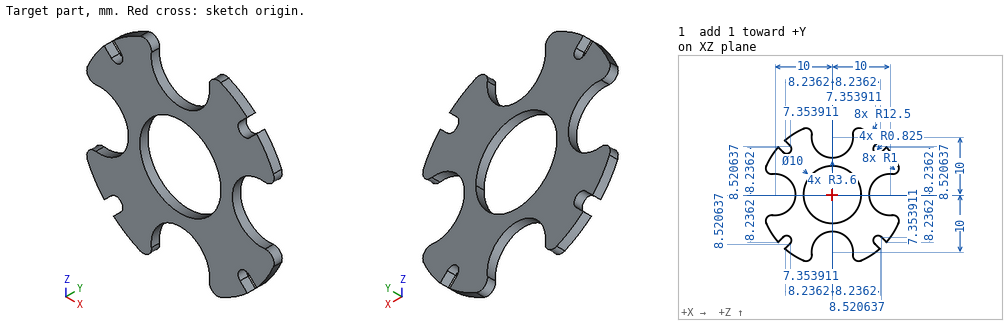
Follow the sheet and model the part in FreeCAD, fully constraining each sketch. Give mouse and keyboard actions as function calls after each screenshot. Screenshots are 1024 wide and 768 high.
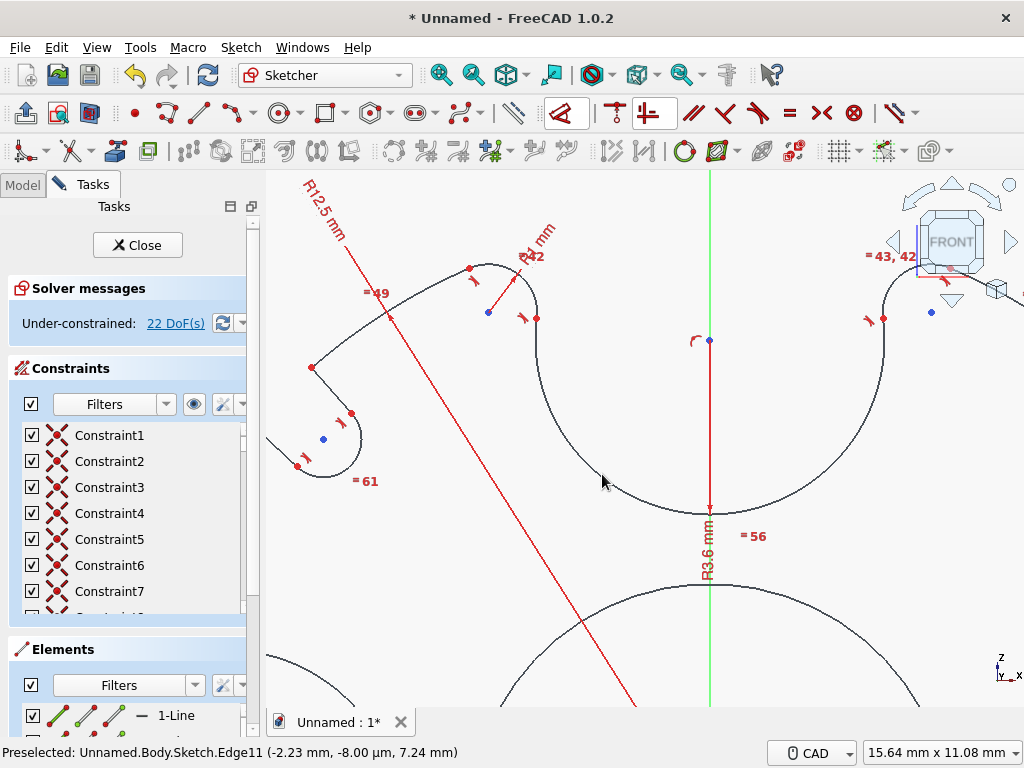
scroll(519, 272, down, 6)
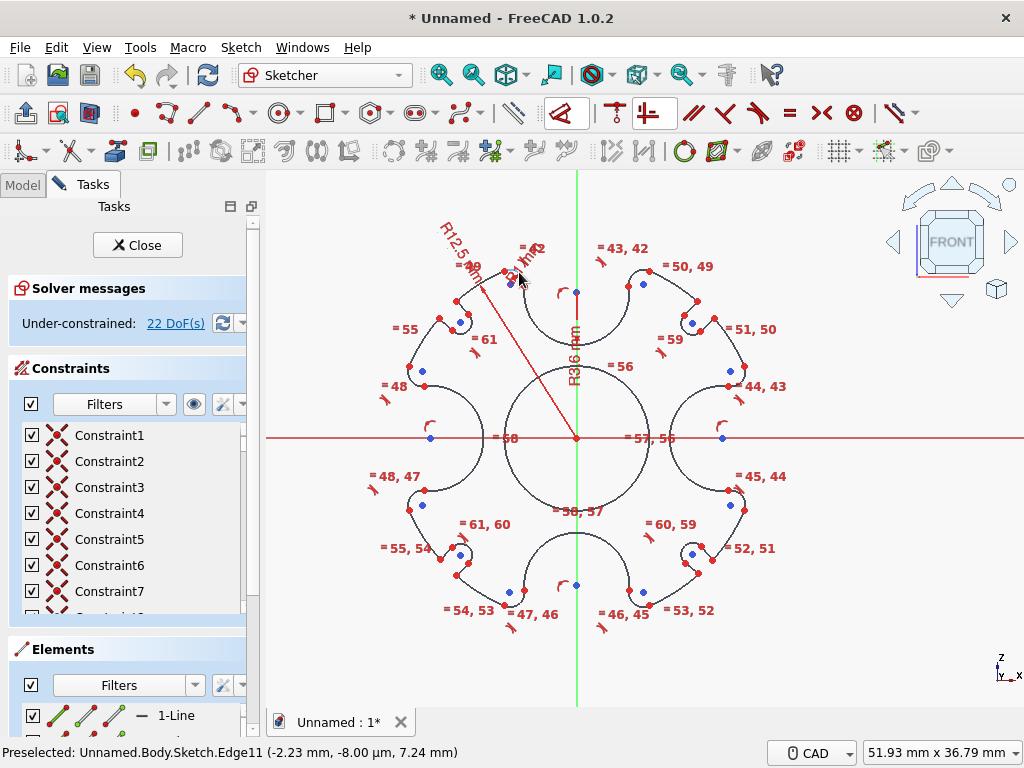
scroll(681, 325, up, 6)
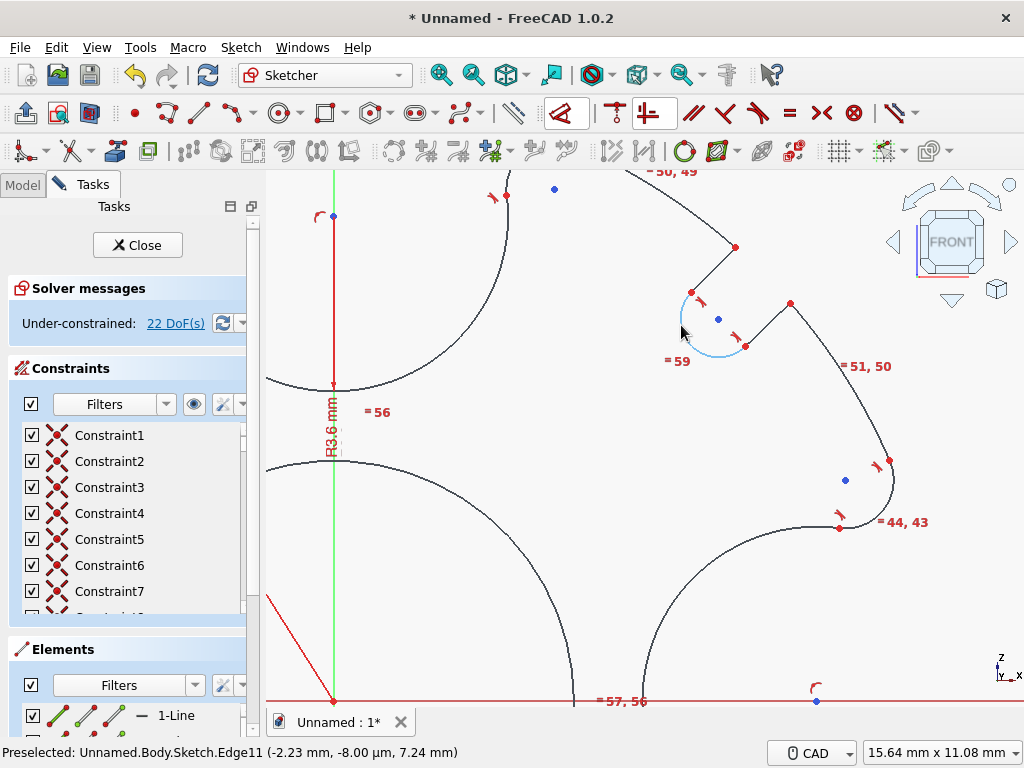
click(681, 325)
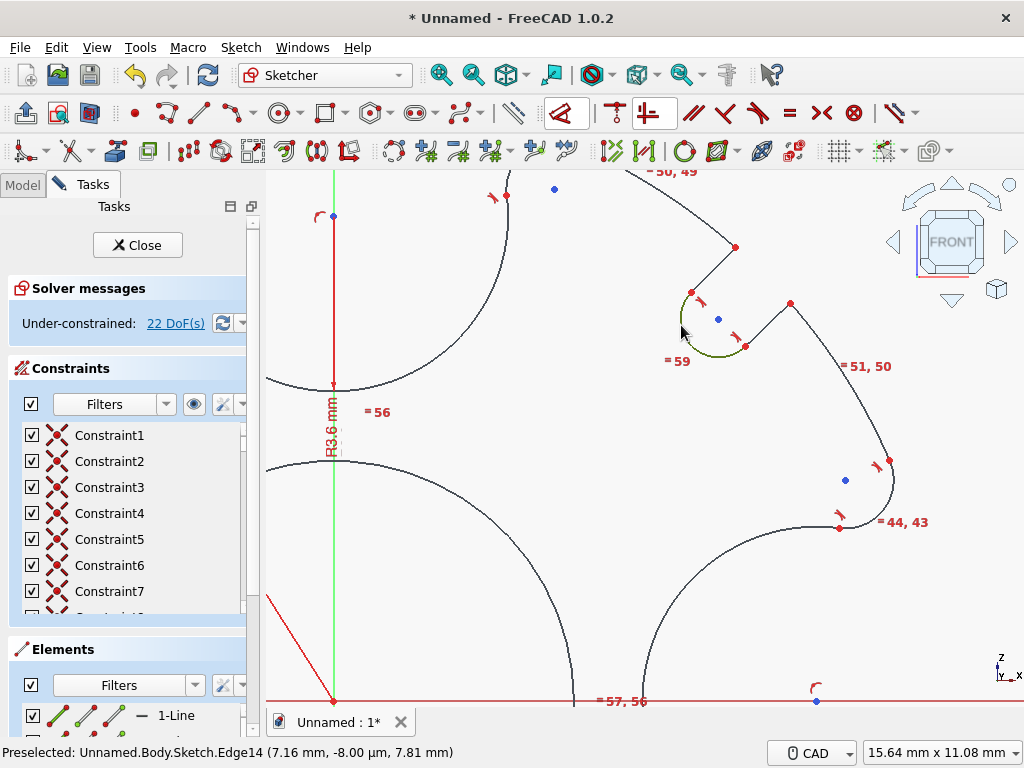
click(584, 114)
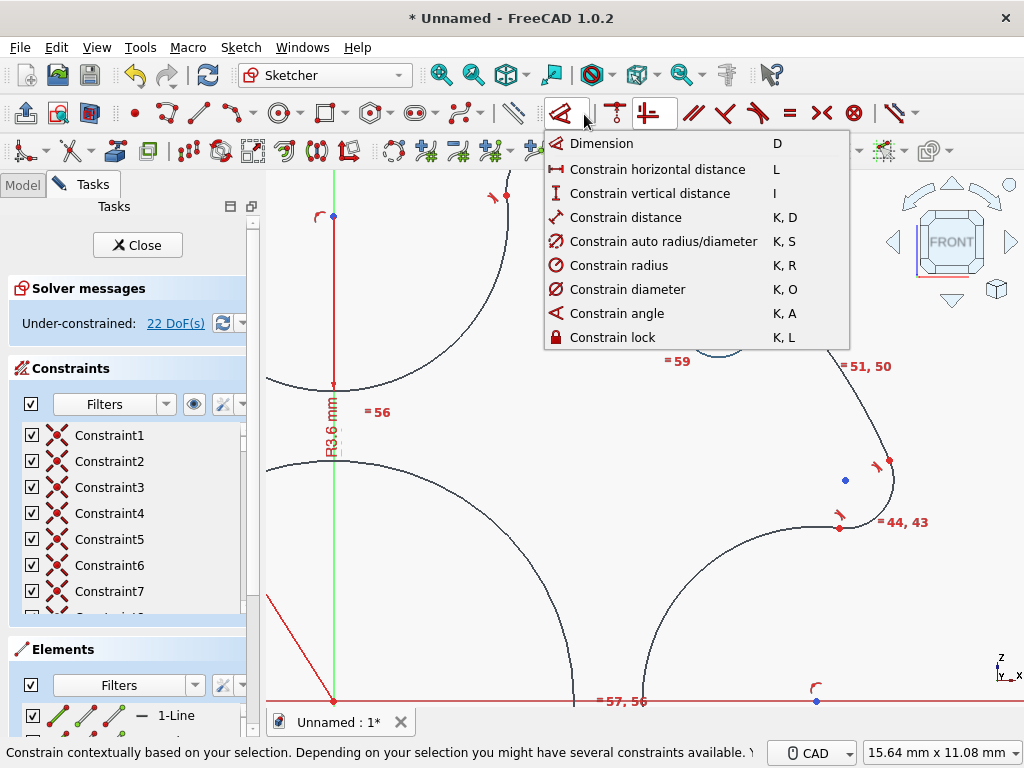
click(697, 265)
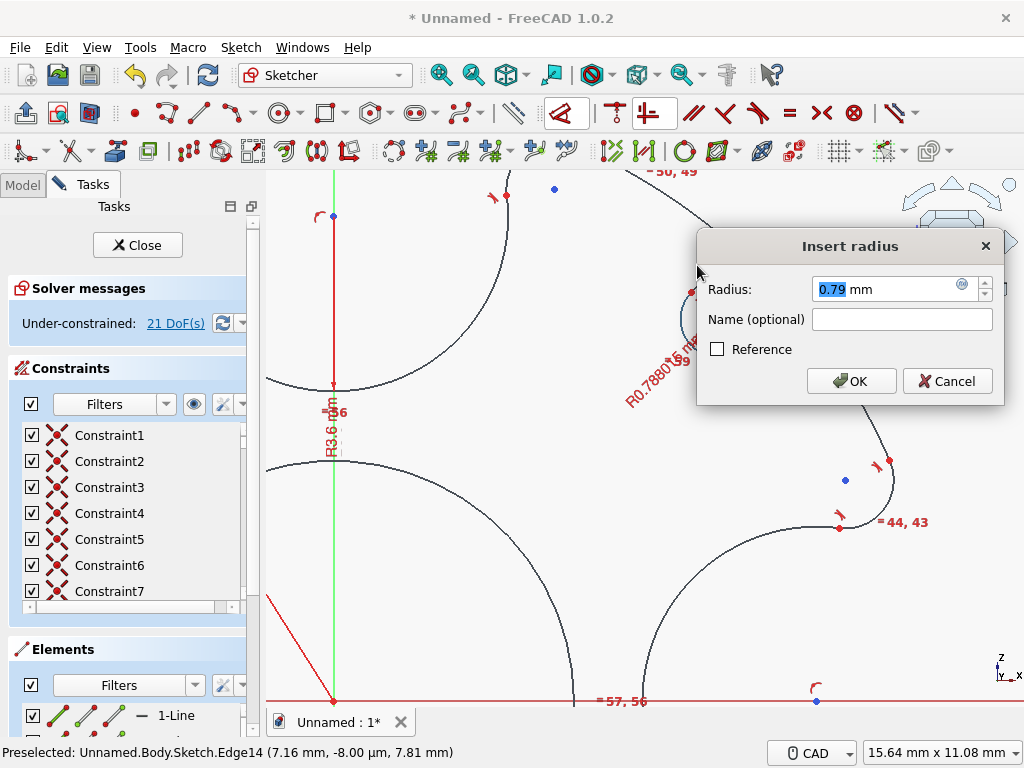
text(0.825)
key(Return)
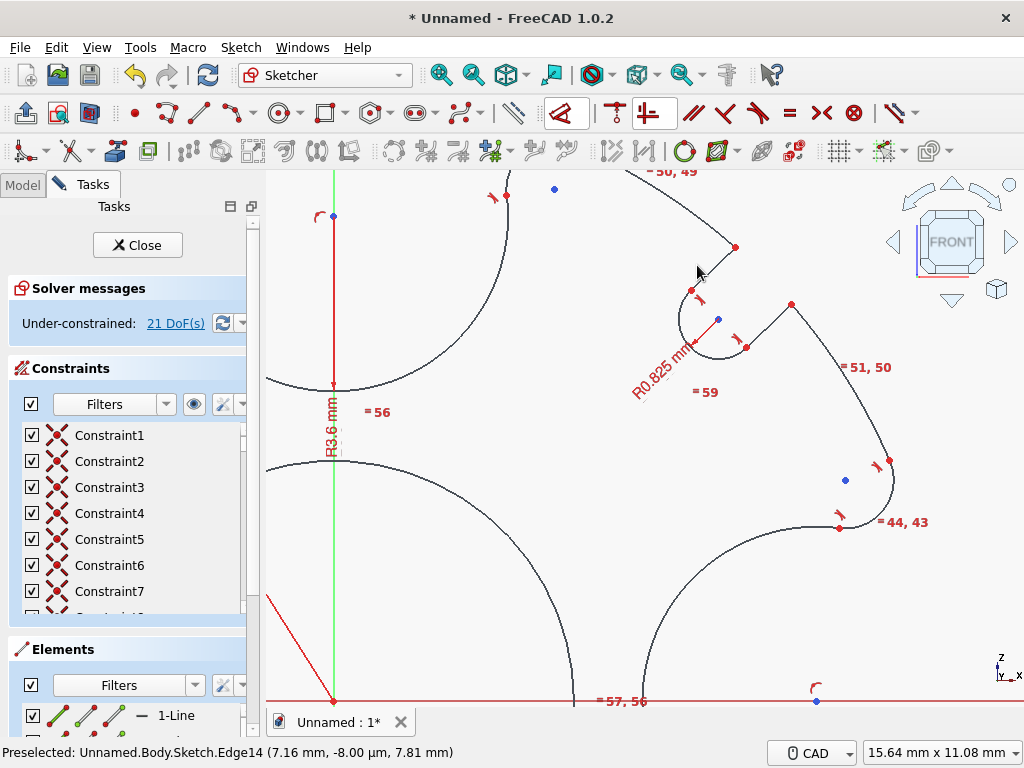
click(503, 531)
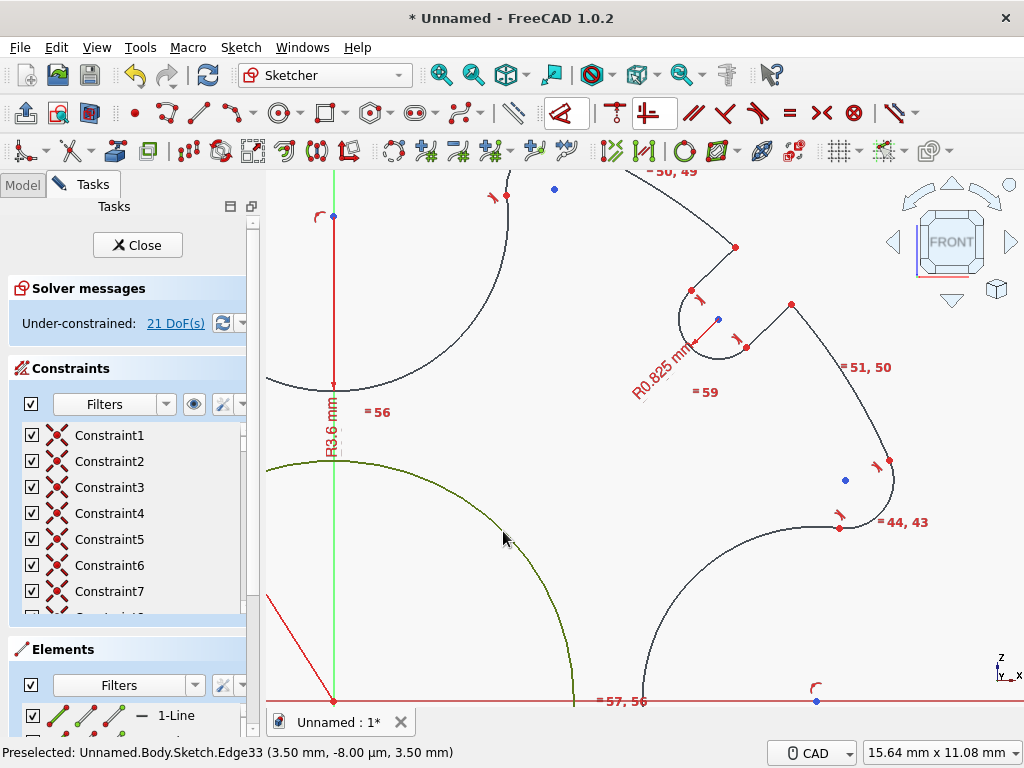
key(k)
key(o)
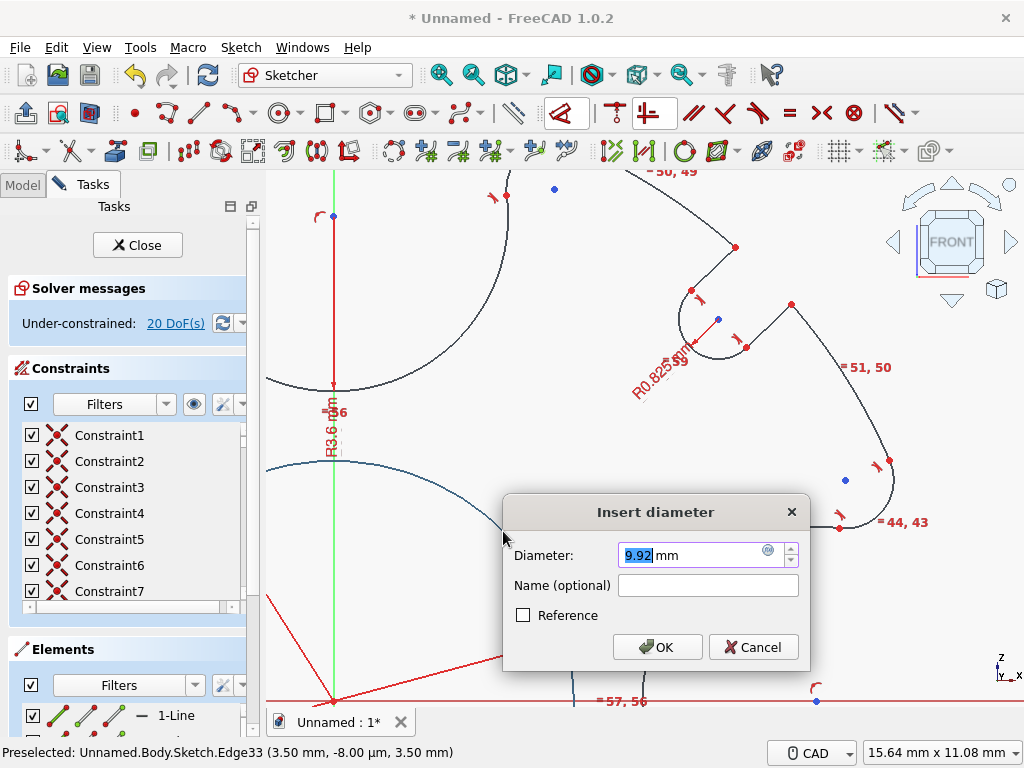
text(10)
key(Return)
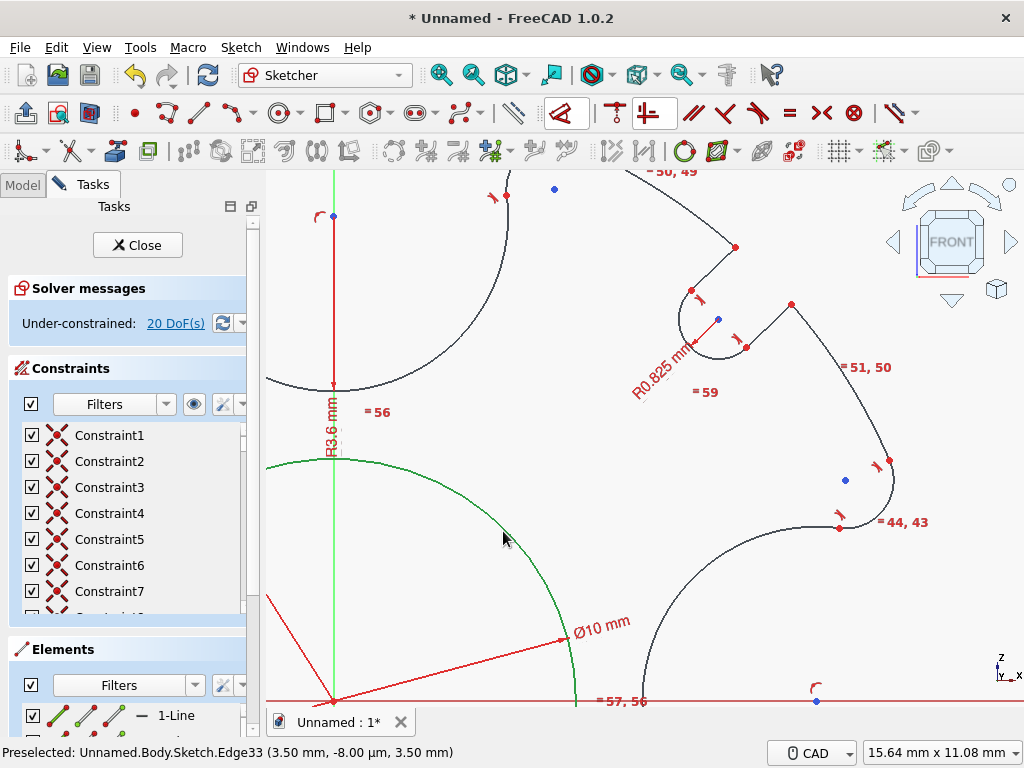
click(334, 217)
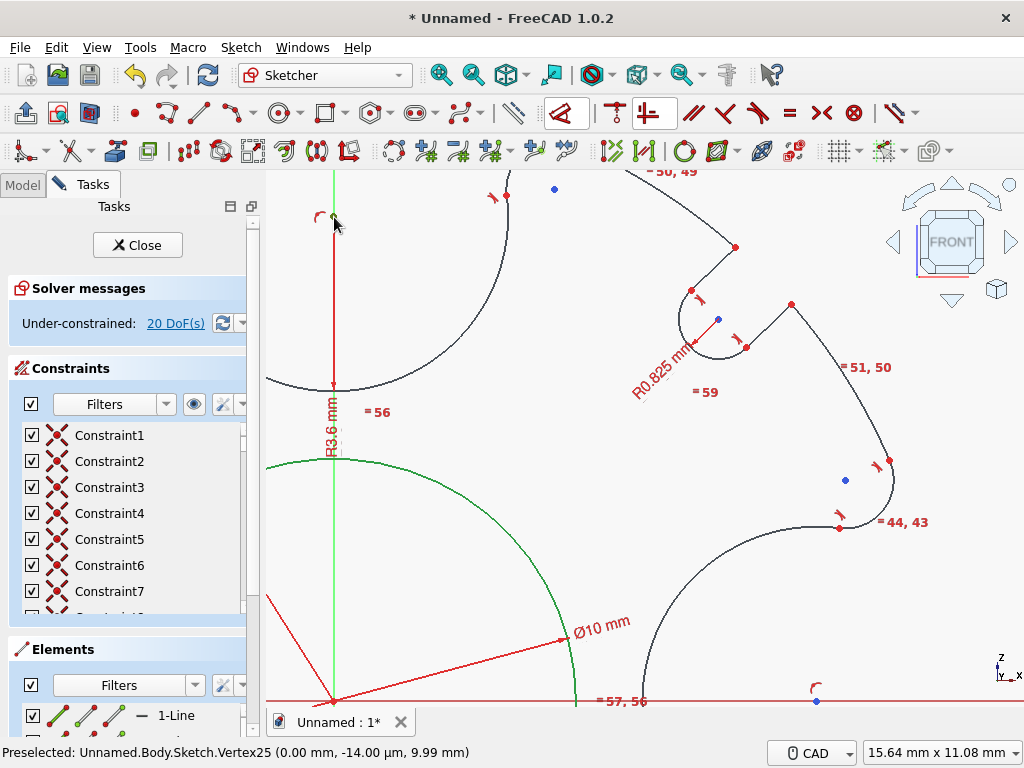
key(i)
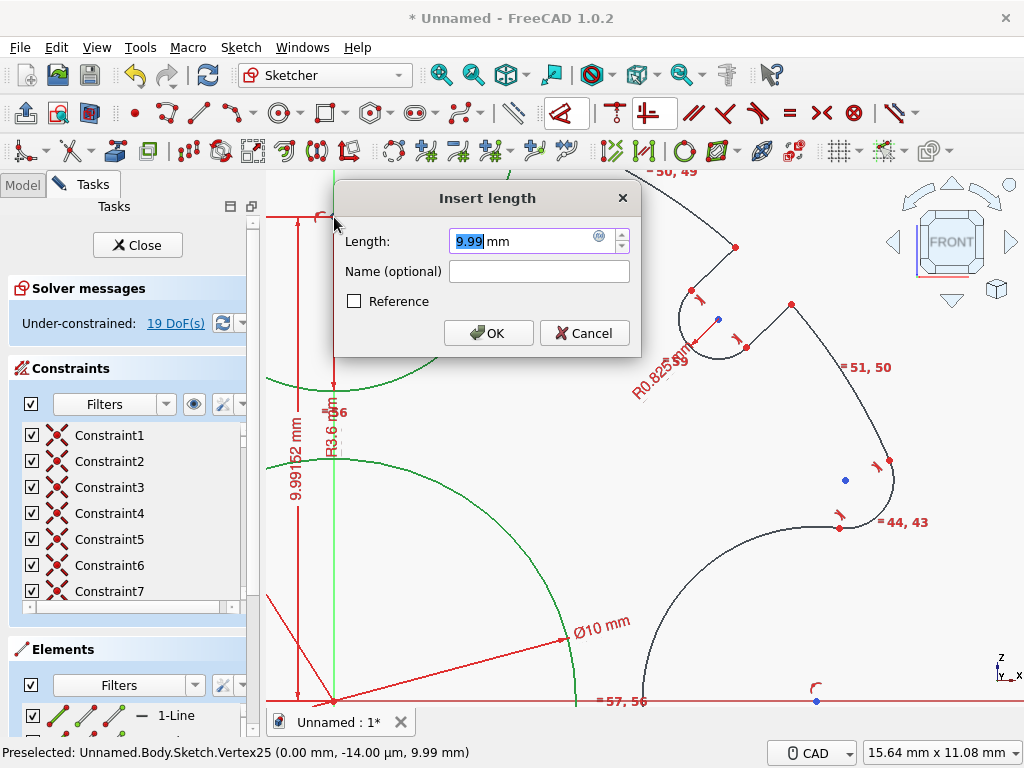
text(10)
key(Return)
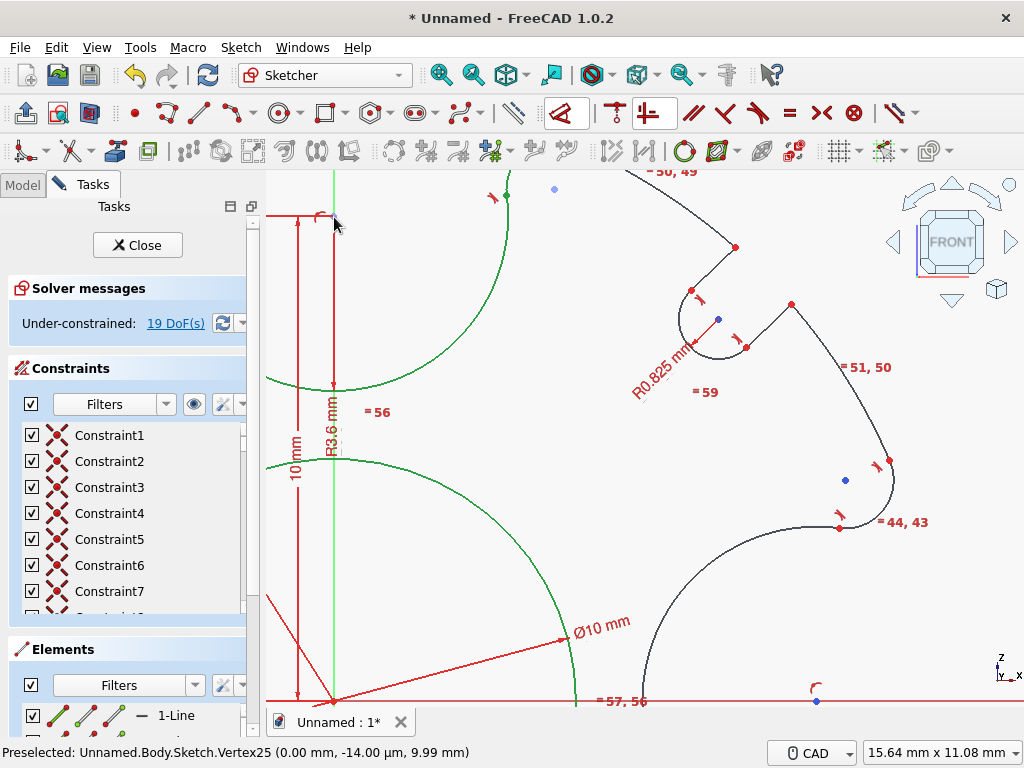
scroll(681, 325, down, 6)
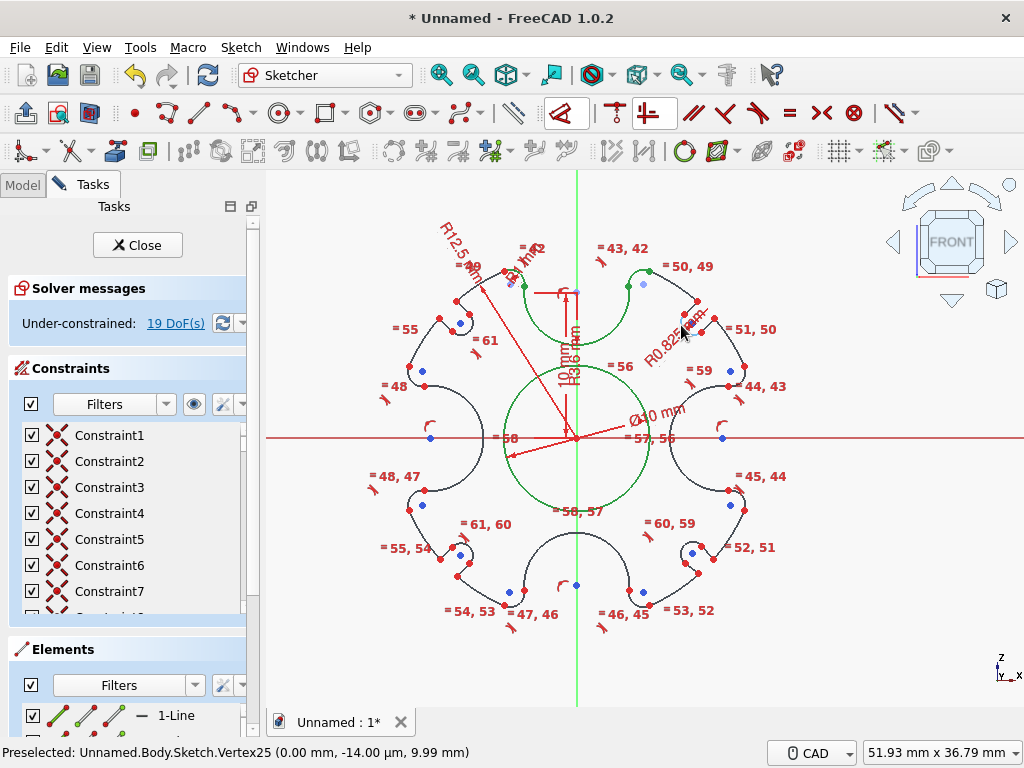
click(722, 438)